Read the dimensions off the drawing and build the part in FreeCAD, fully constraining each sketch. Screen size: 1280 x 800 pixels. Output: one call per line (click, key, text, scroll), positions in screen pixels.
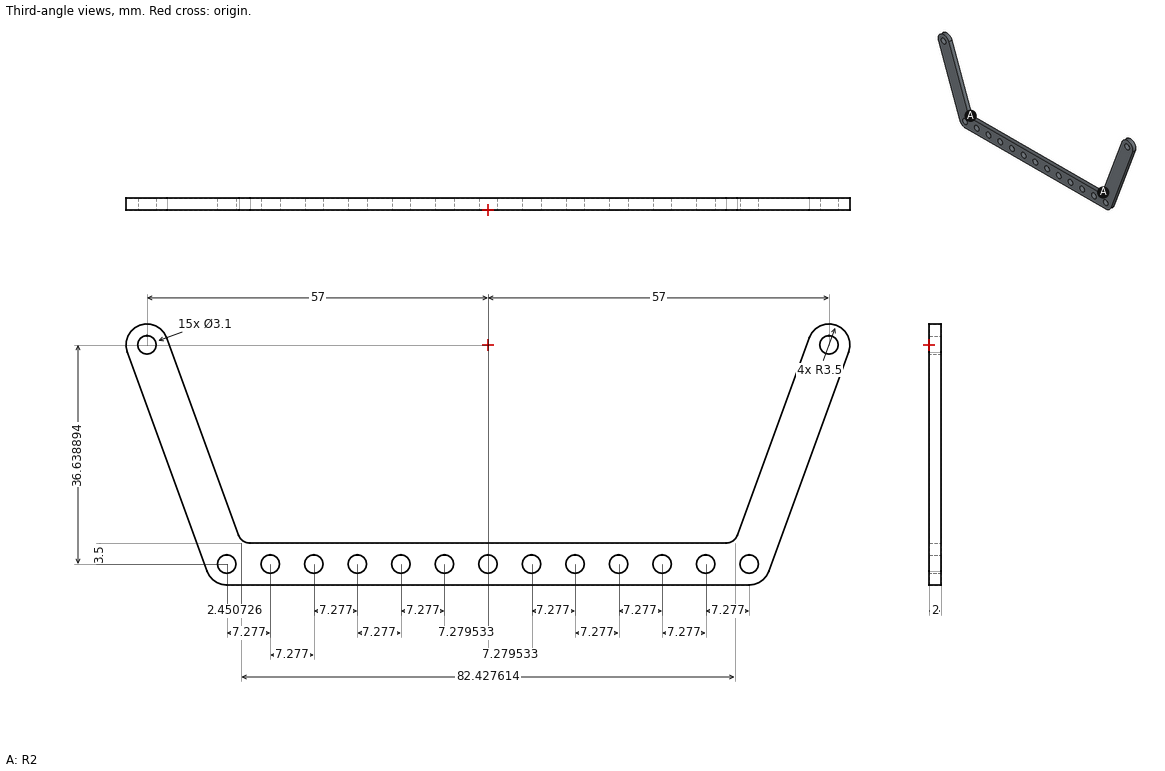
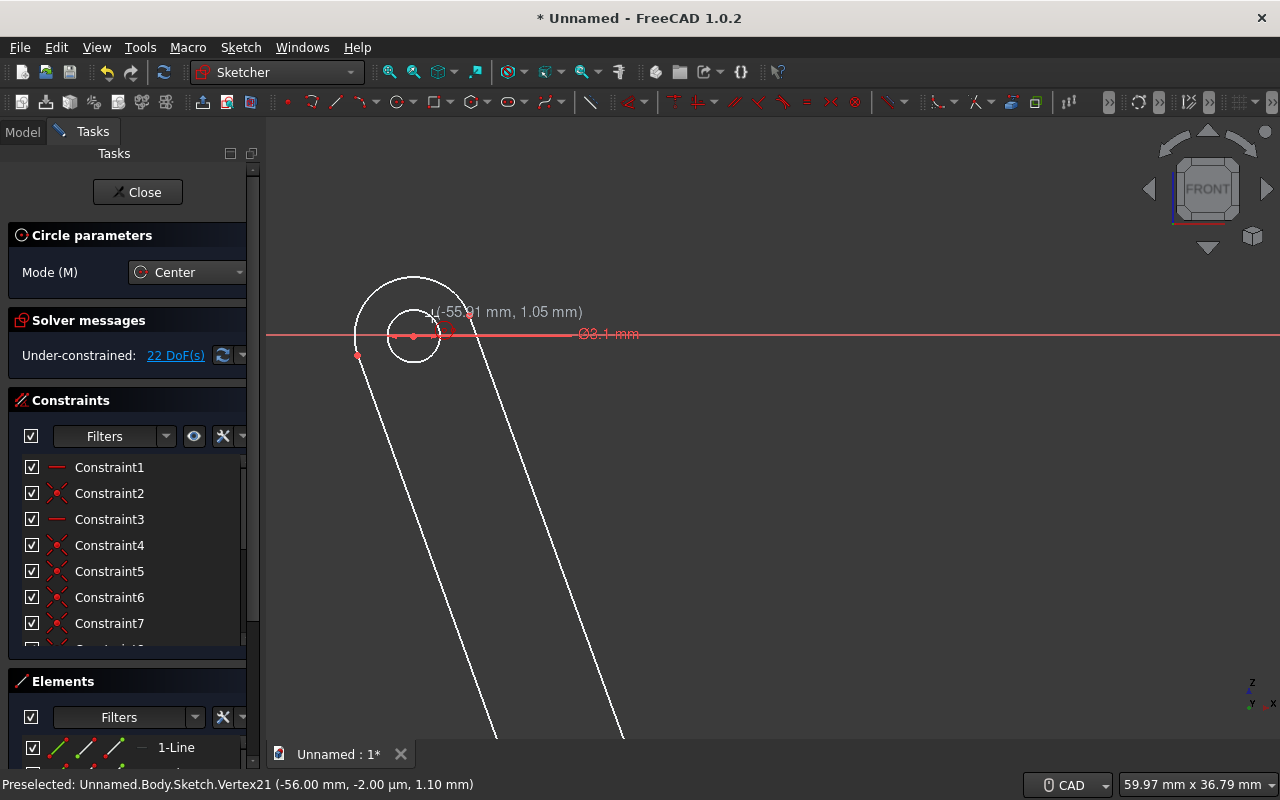
scroll(414, 334, down, 6)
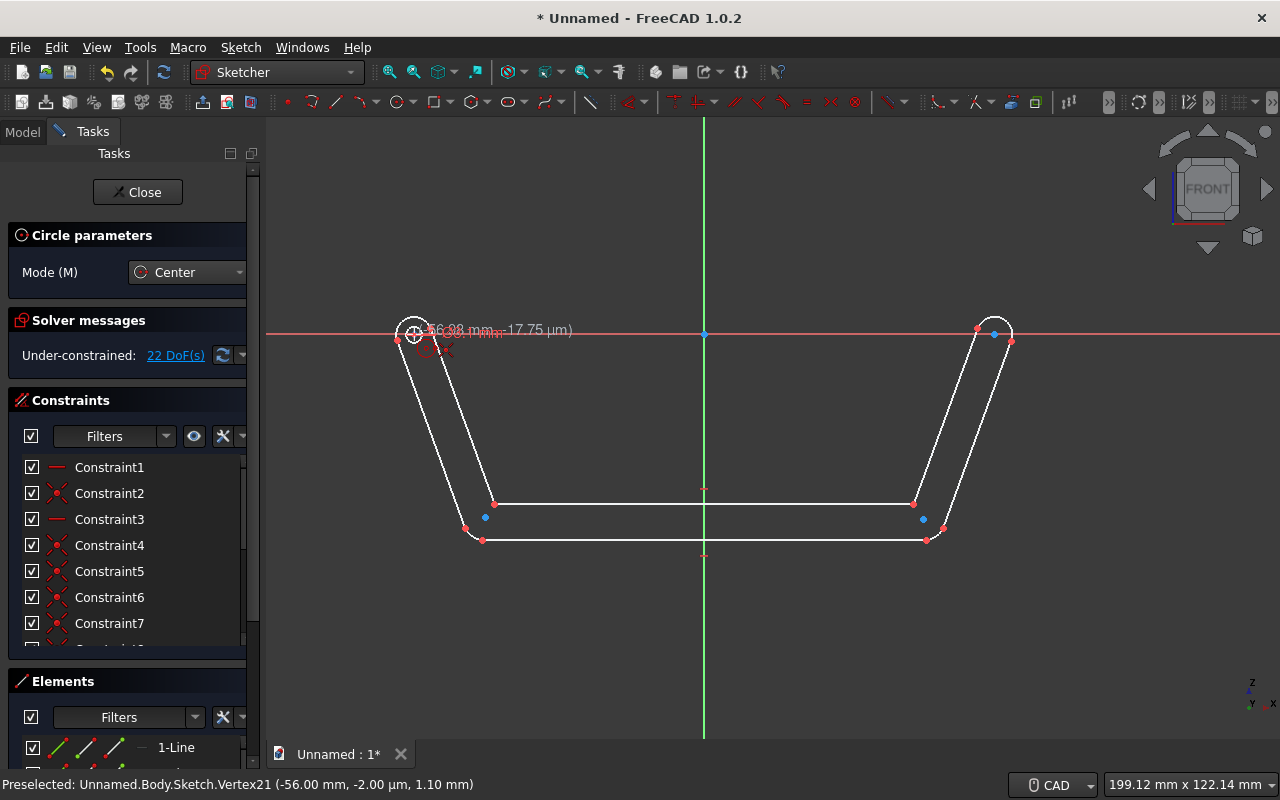
scroll(995, 334, up, 6)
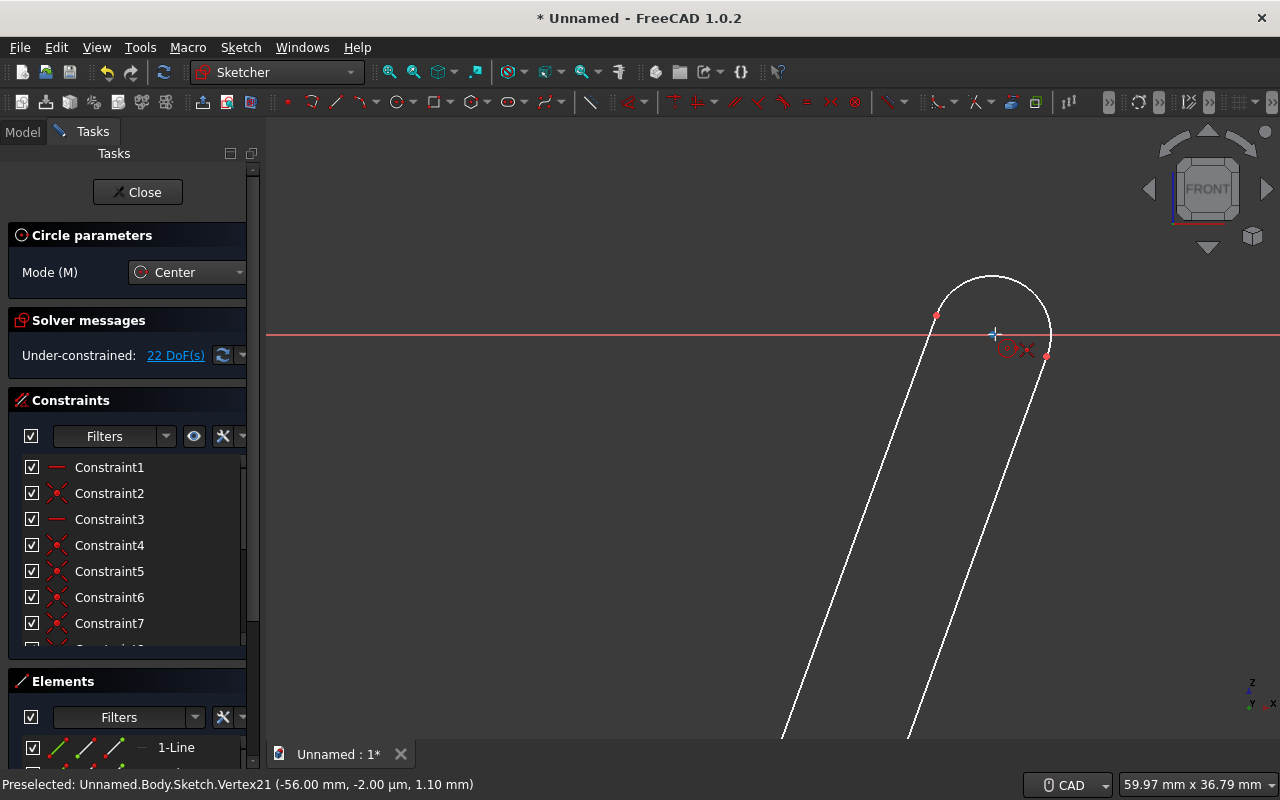
click(992, 335)
move(1010, 316)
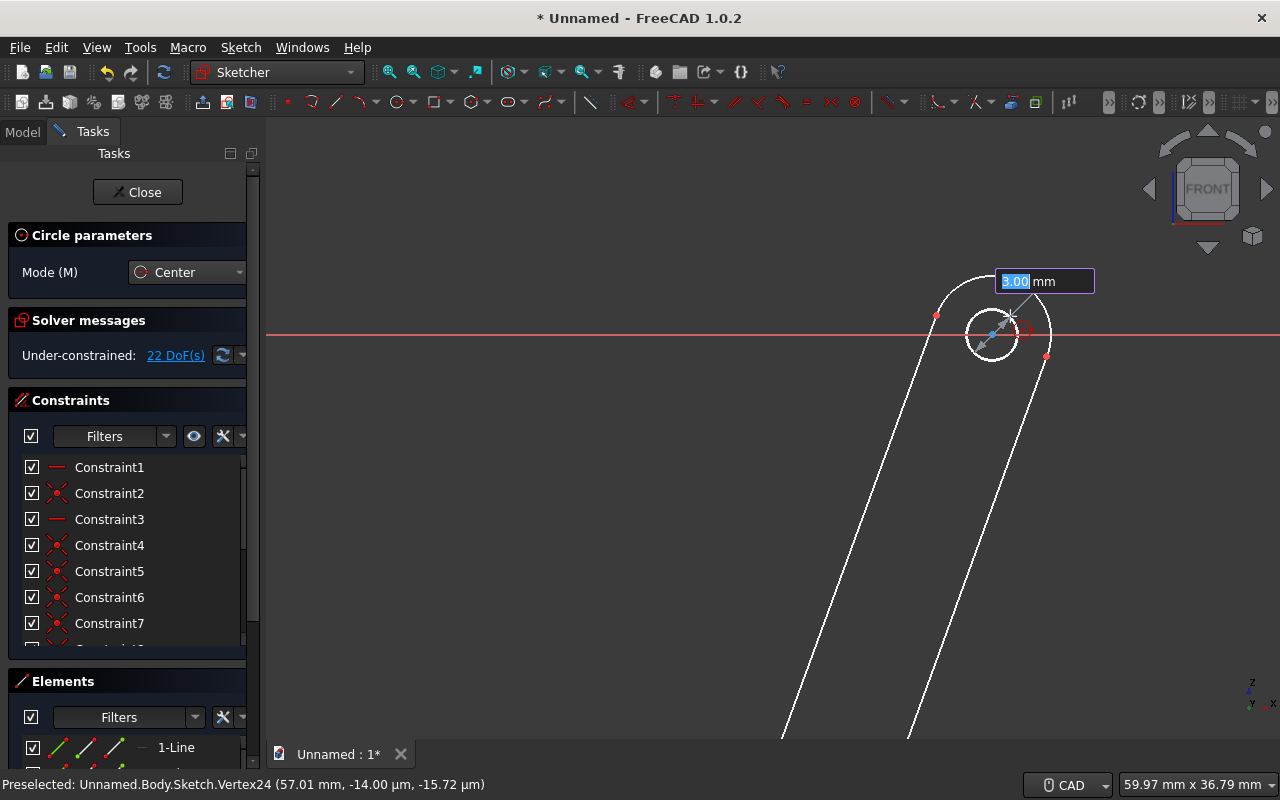
text(3.1)
key(Return)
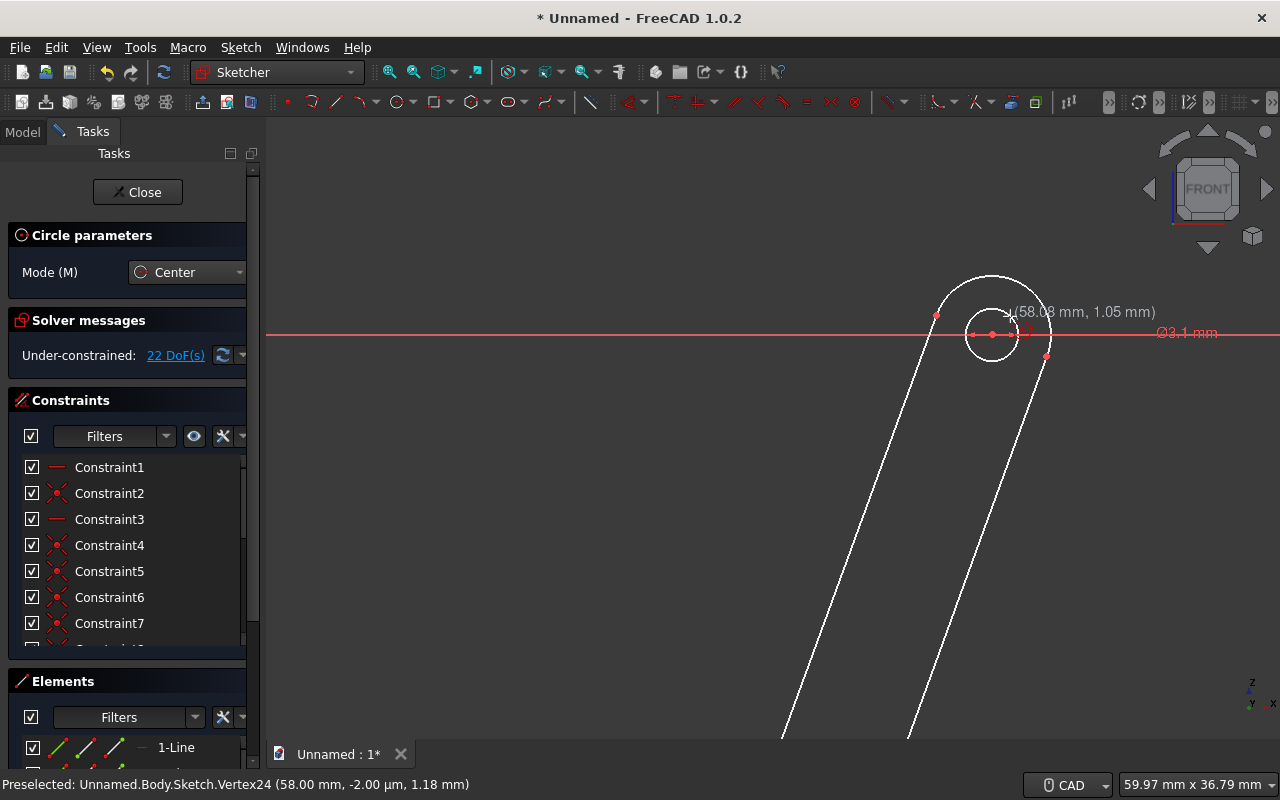
scroll(996, 334, down, 6)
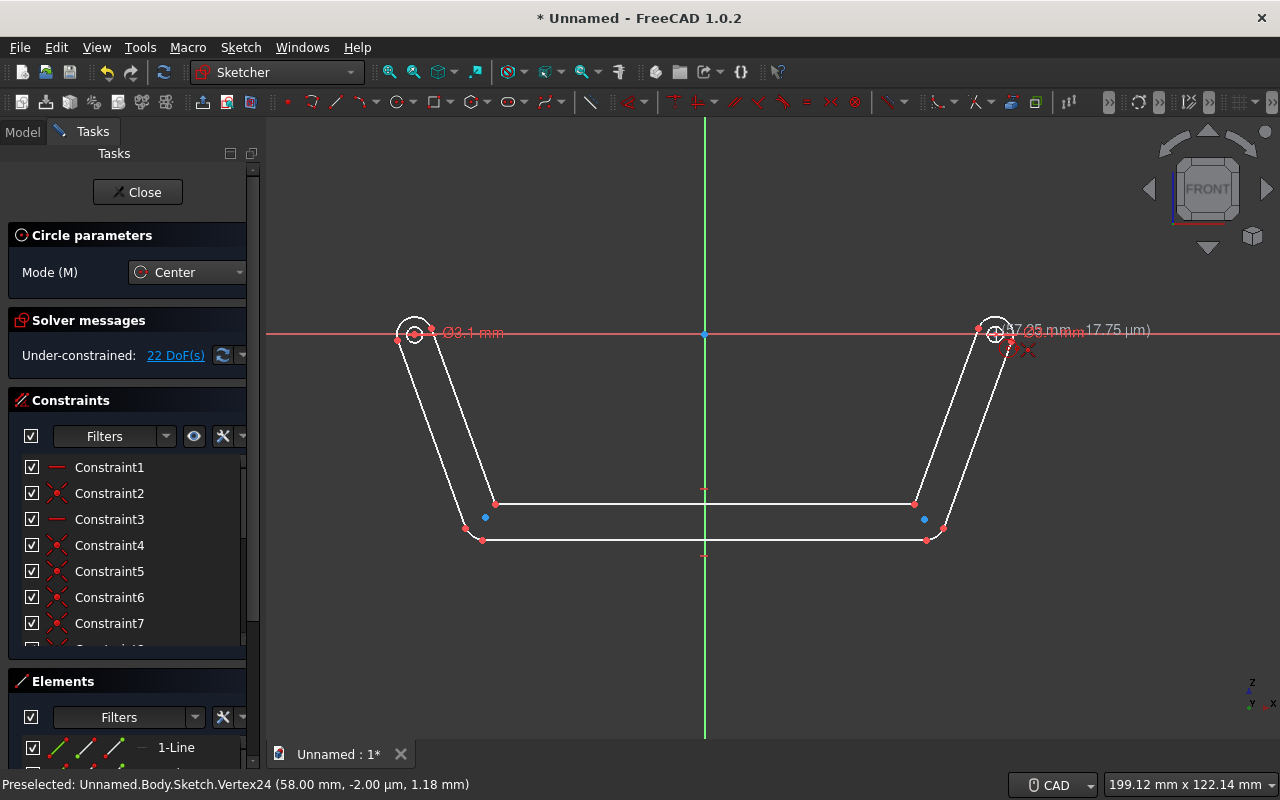
scroll(483, 521, up, 6)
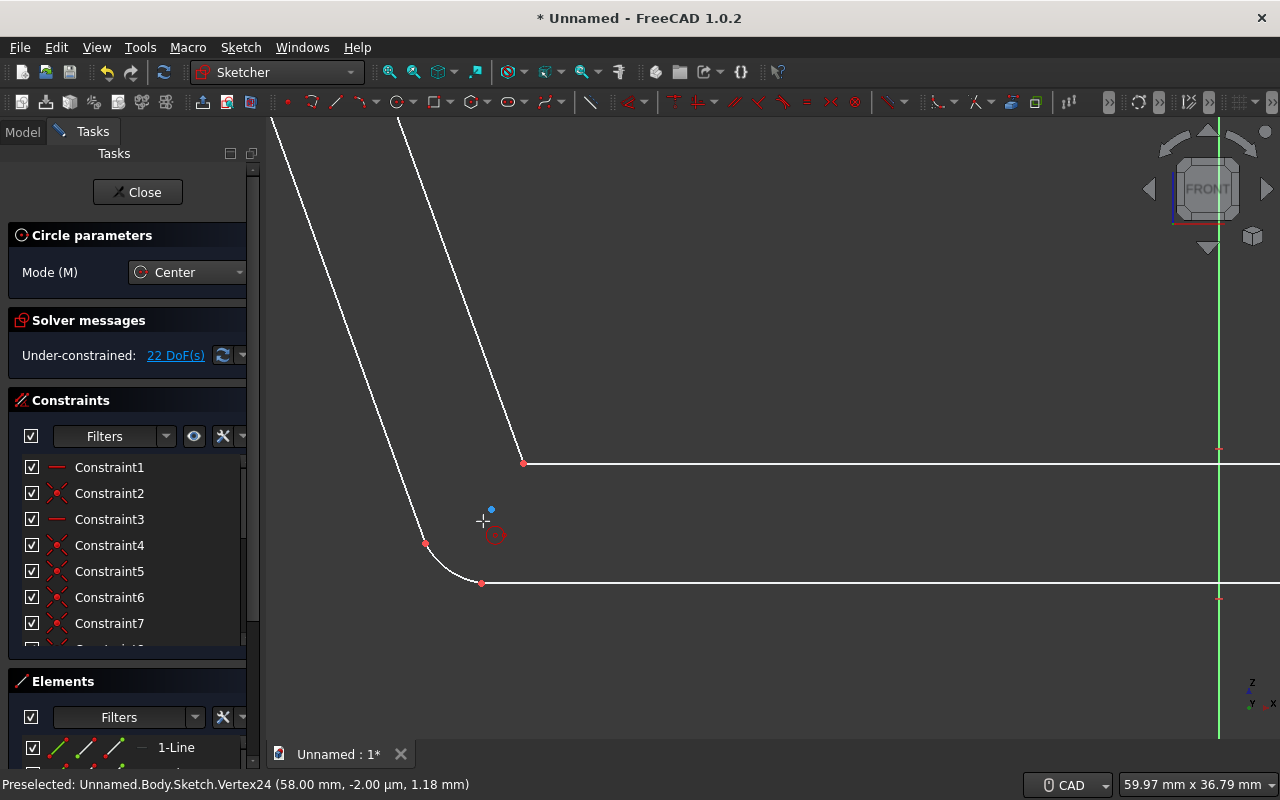
click(481, 520)
move(500, 501)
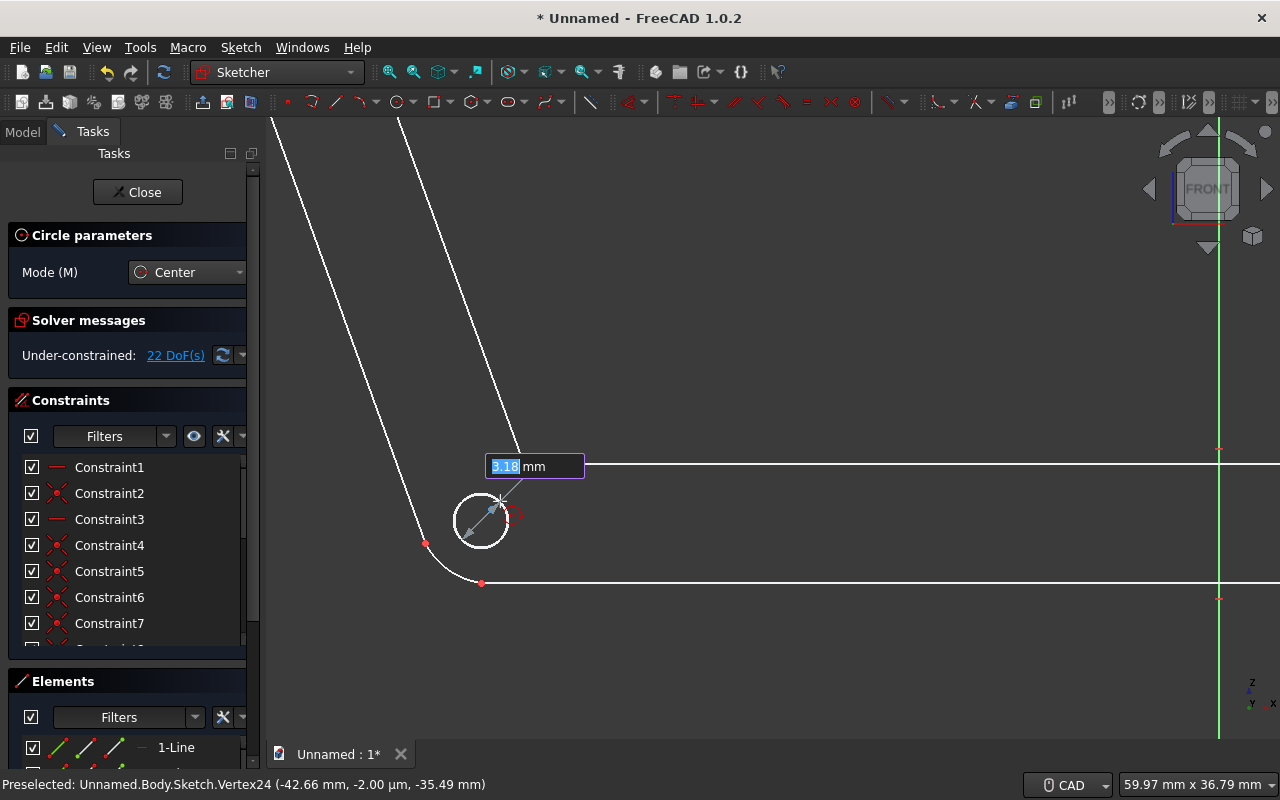
text(3.1)
key(Return)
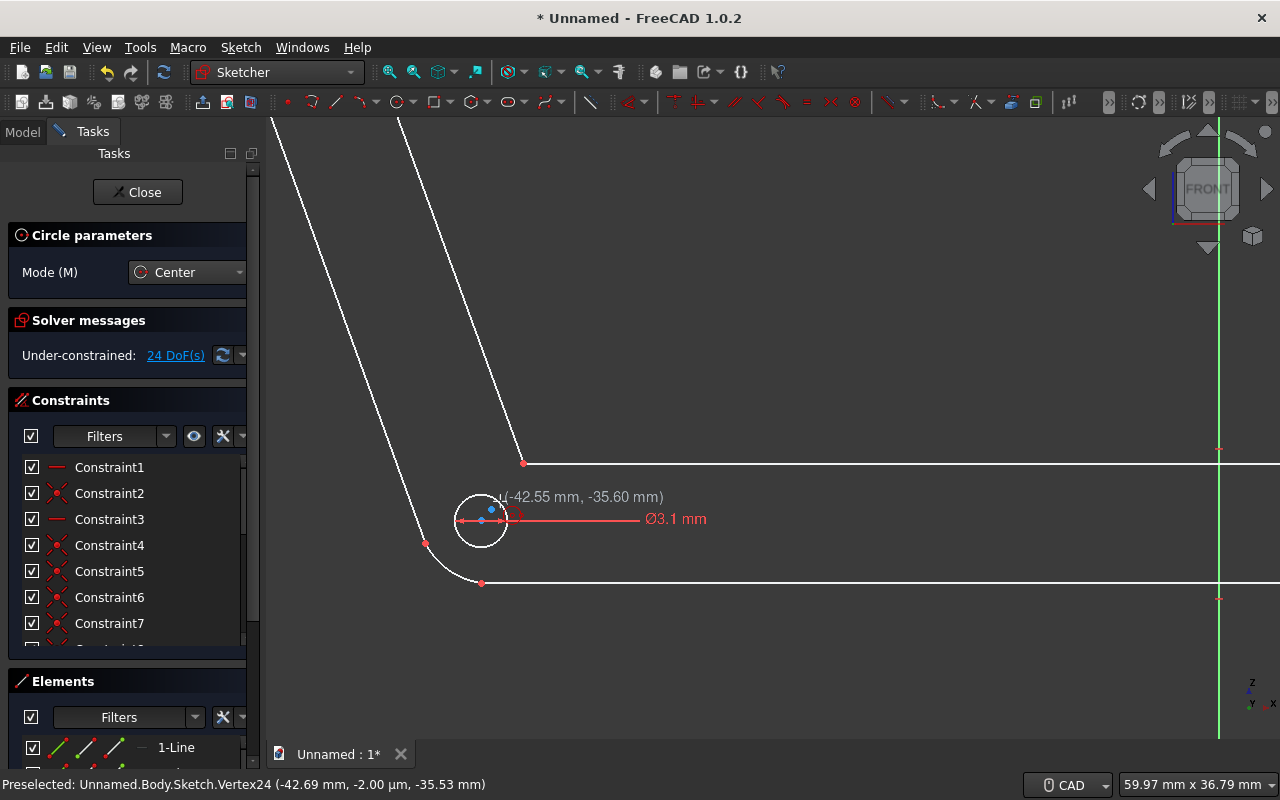
click(604, 520)
move(623, 501)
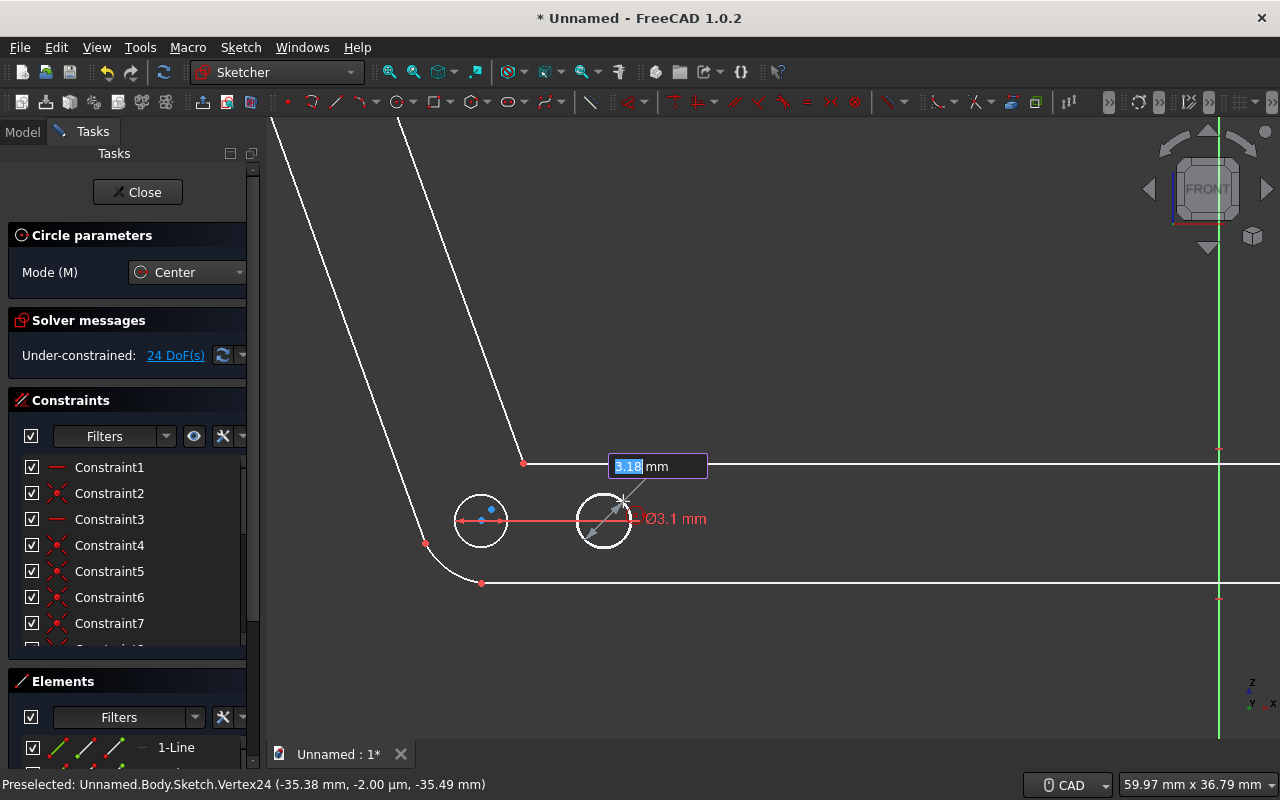
text(3.1)
key(Return)